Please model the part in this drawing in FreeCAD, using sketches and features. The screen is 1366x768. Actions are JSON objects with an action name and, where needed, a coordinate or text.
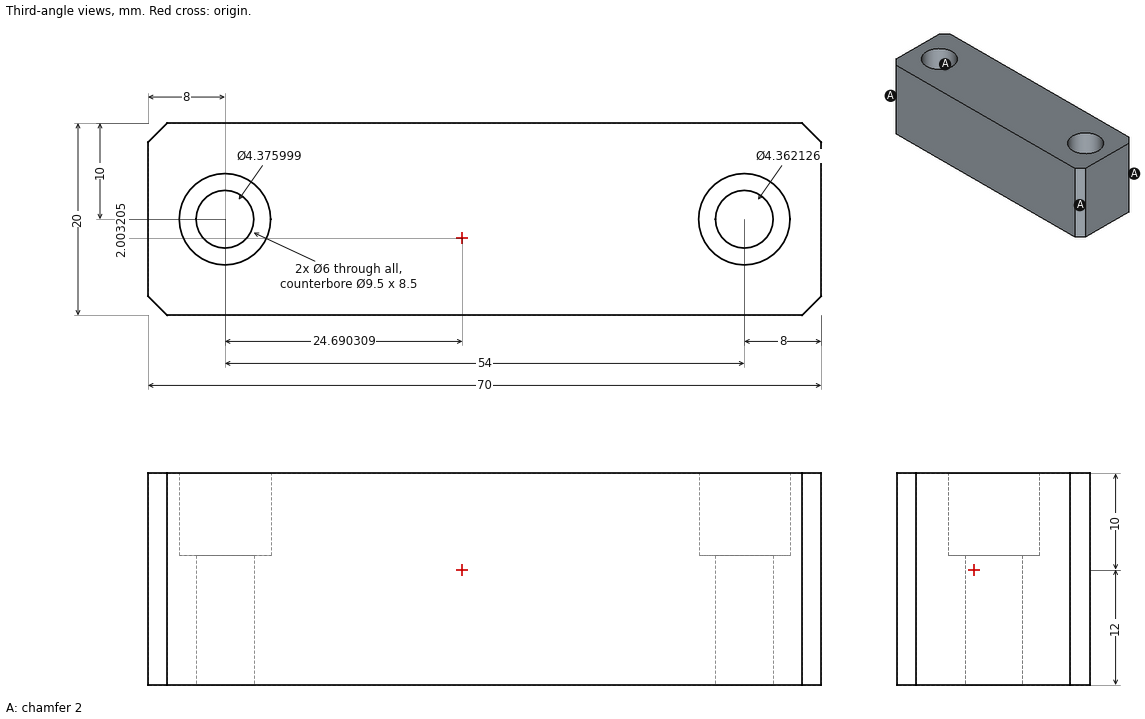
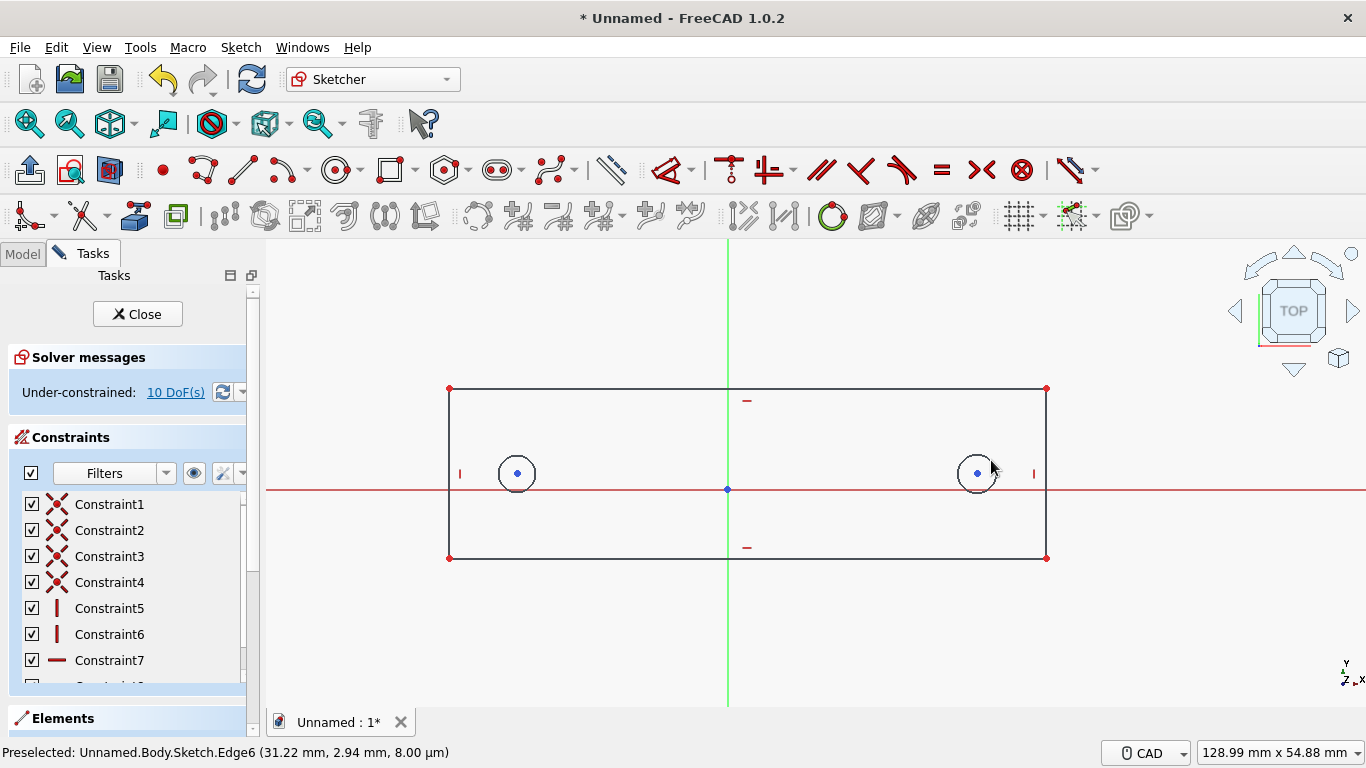
{"action": "left_click", "coordinate": [517, 474]}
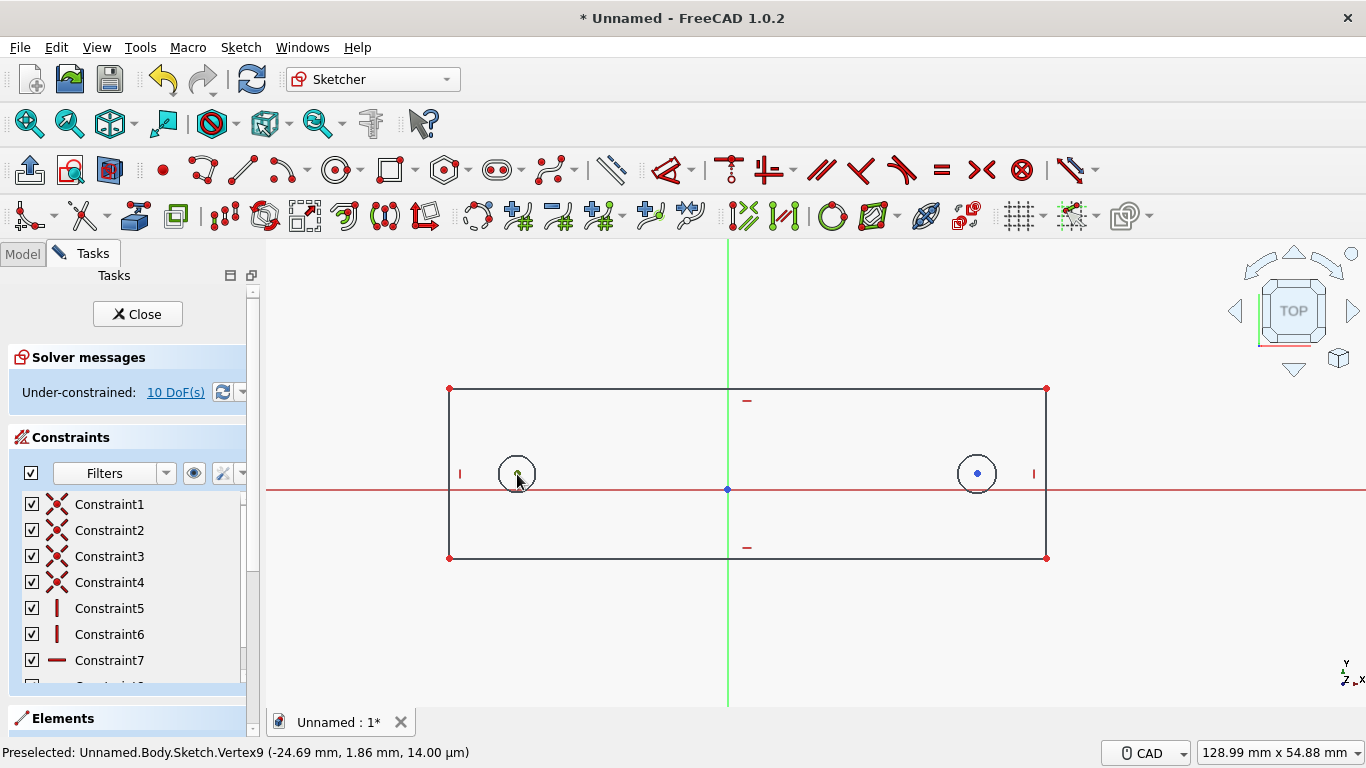
{"action": "left_click", "coordinate": [977, 474]}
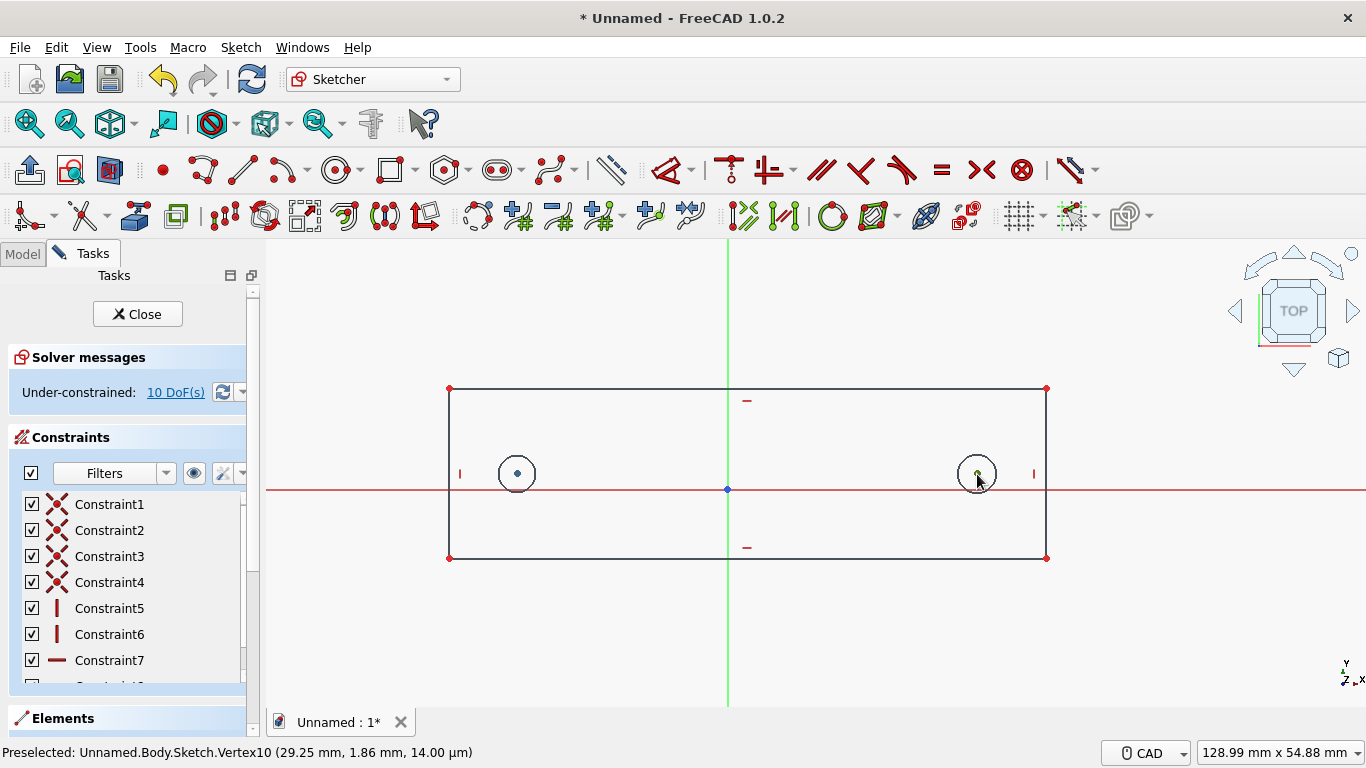
{"action": "key", "text": "h"}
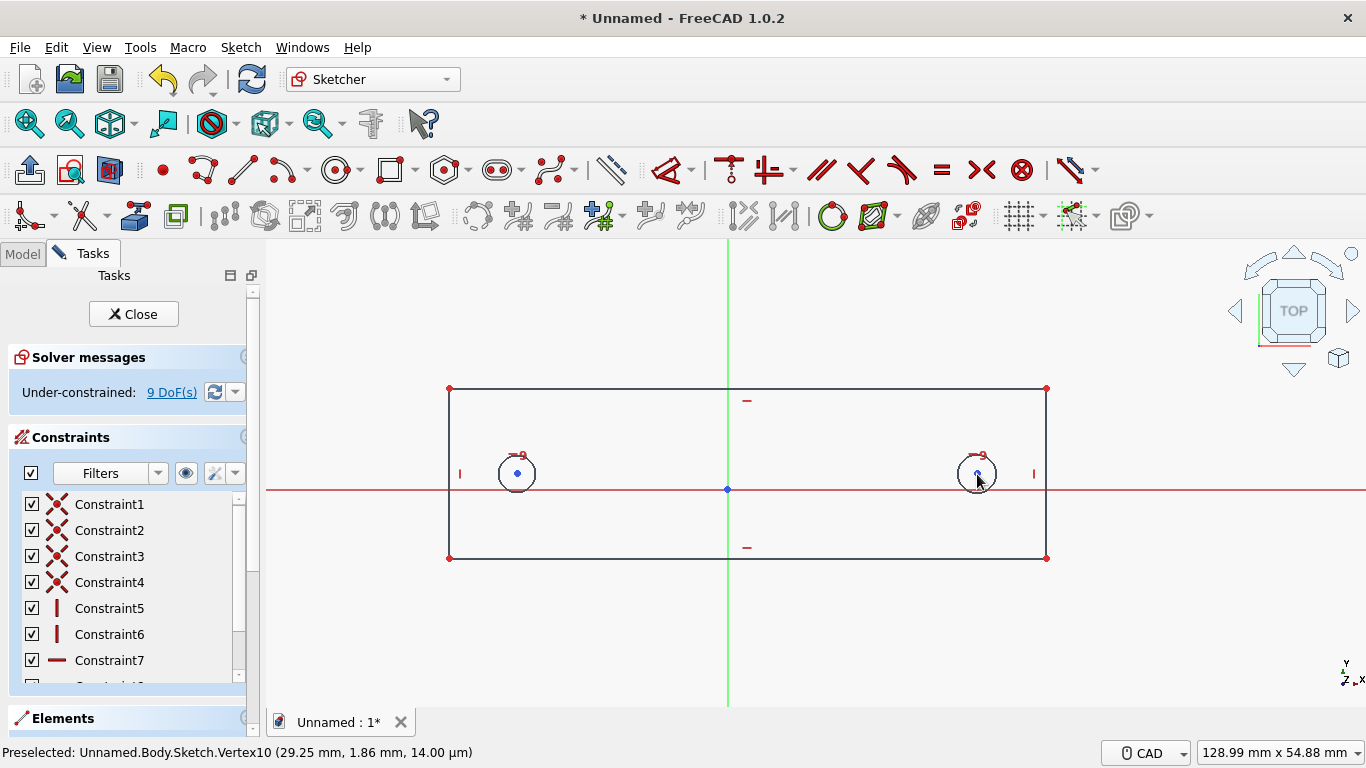
{"action": "left_click", "coordinate": [530, 461]}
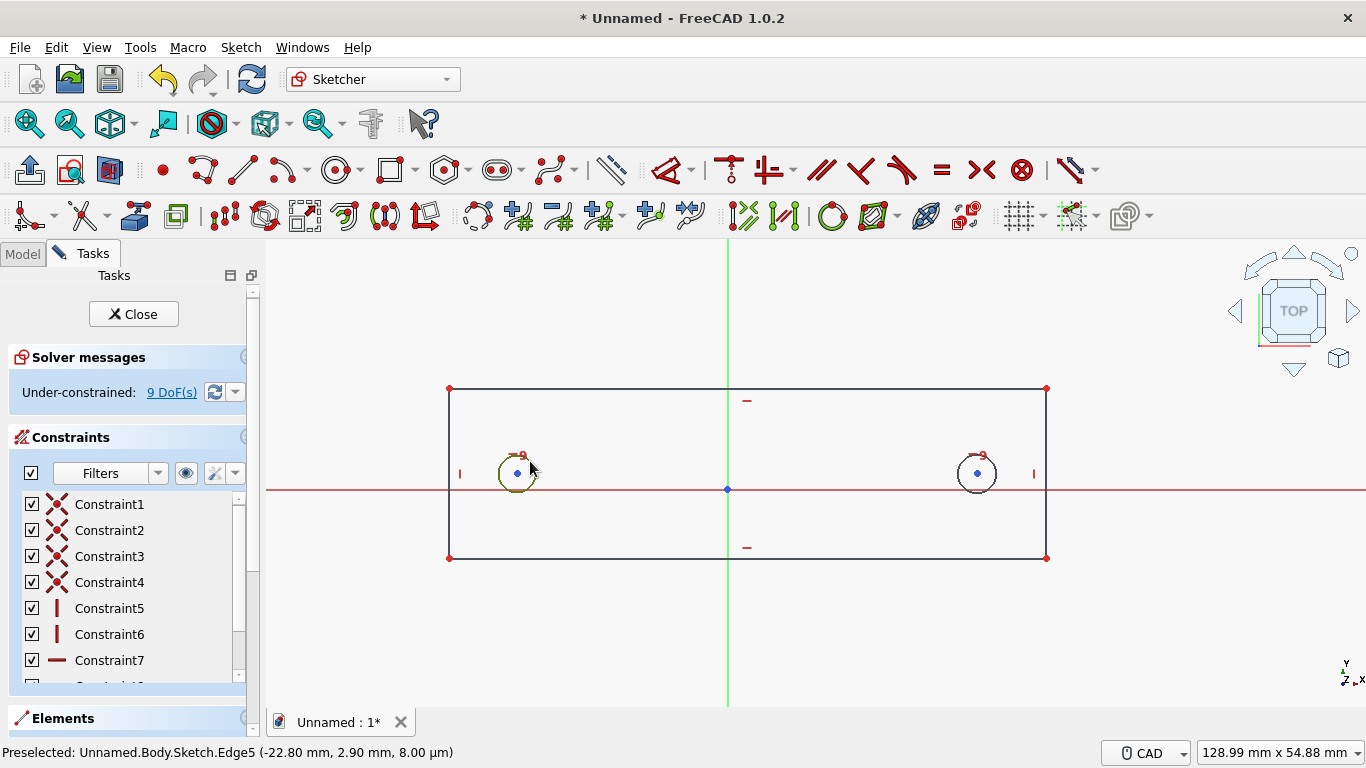
{"action": "key", "text": "k o"}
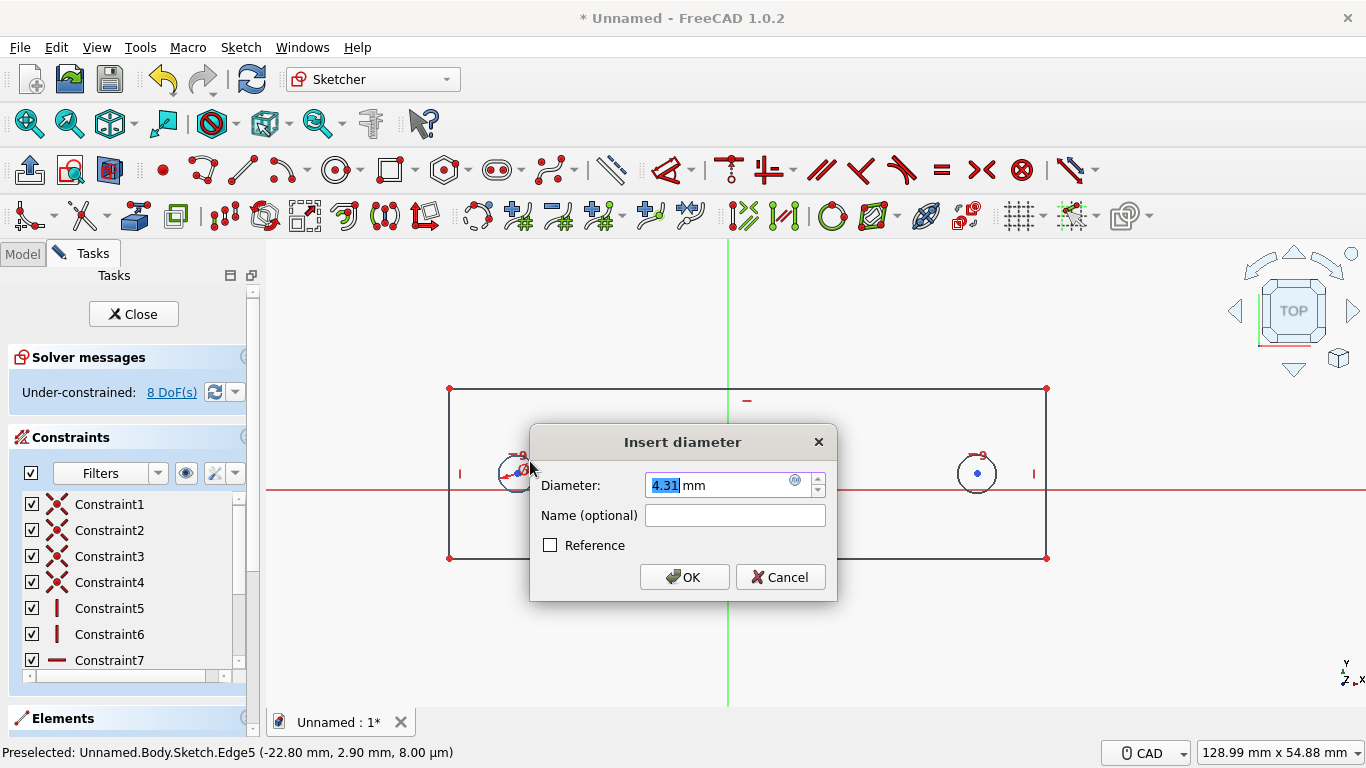
{"action": "type", "text": "4.375999"}
{"action": "key", "text": "Return"}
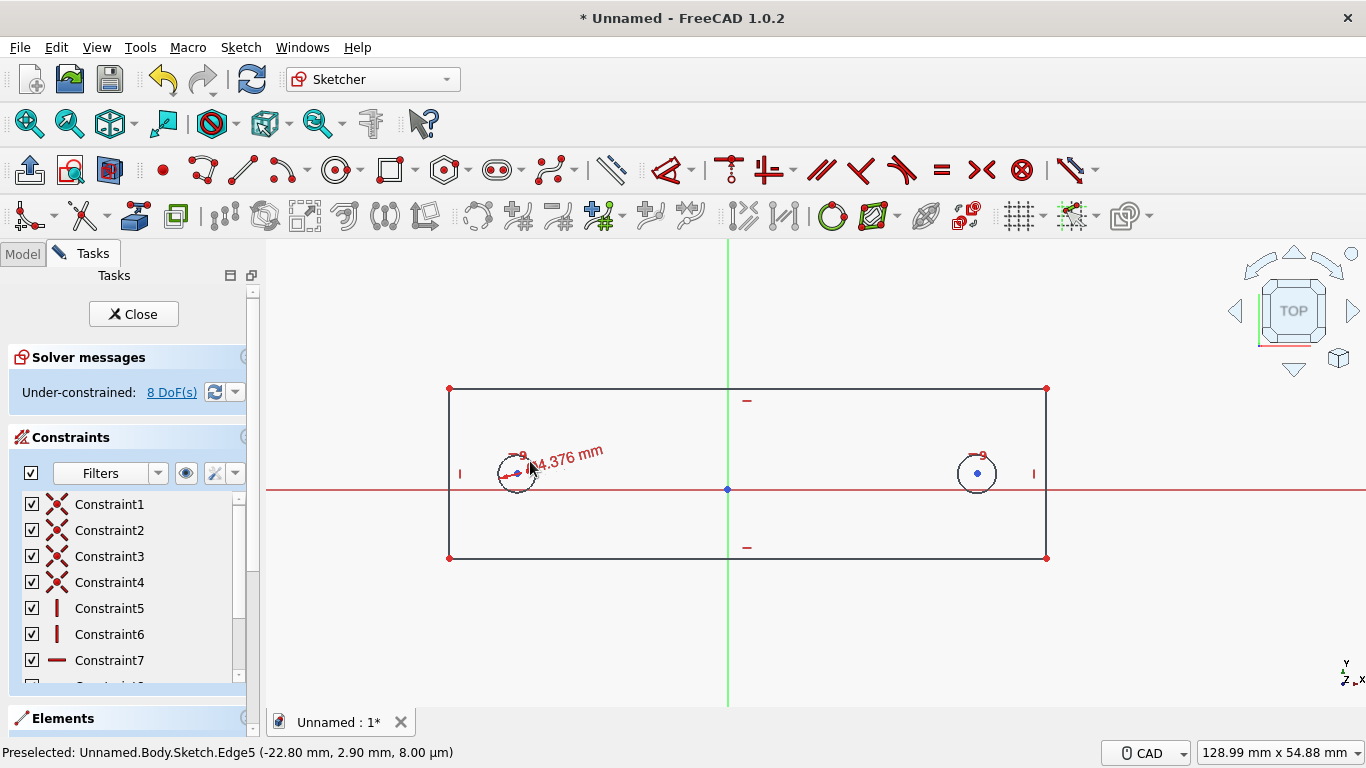
{"action": "left_click", "coordinate": [990, 460]}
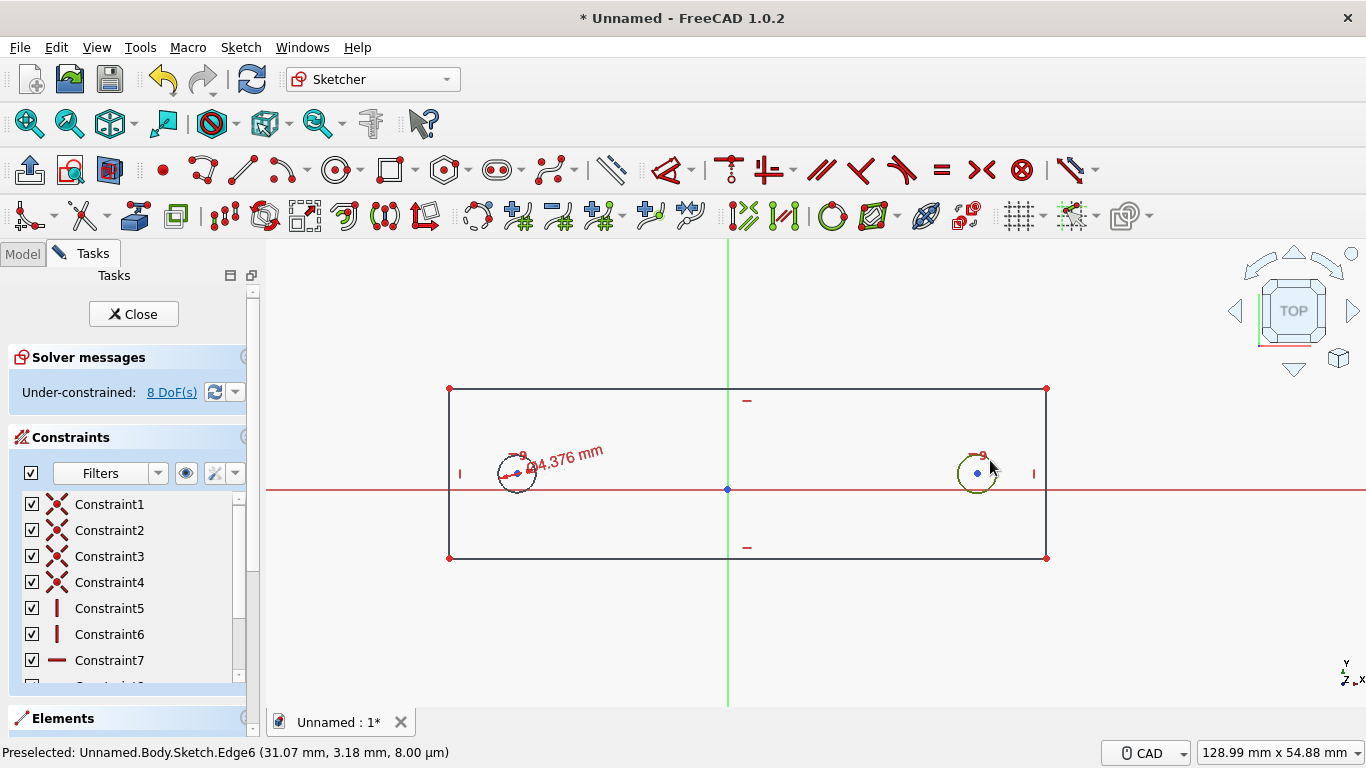
{"action": "key", "text": "k o"}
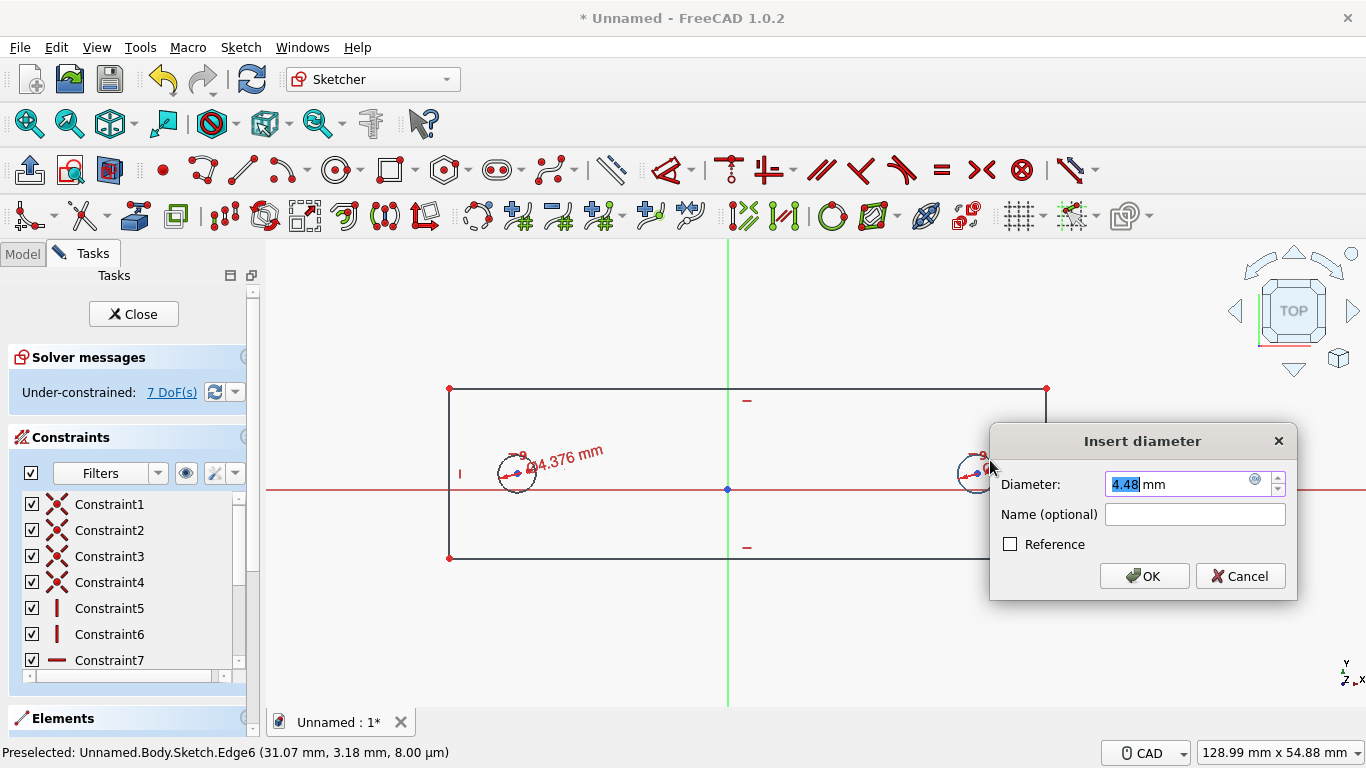
{"action": "type", "text": "4.362126"}
{"action": "key", "text": "Return"}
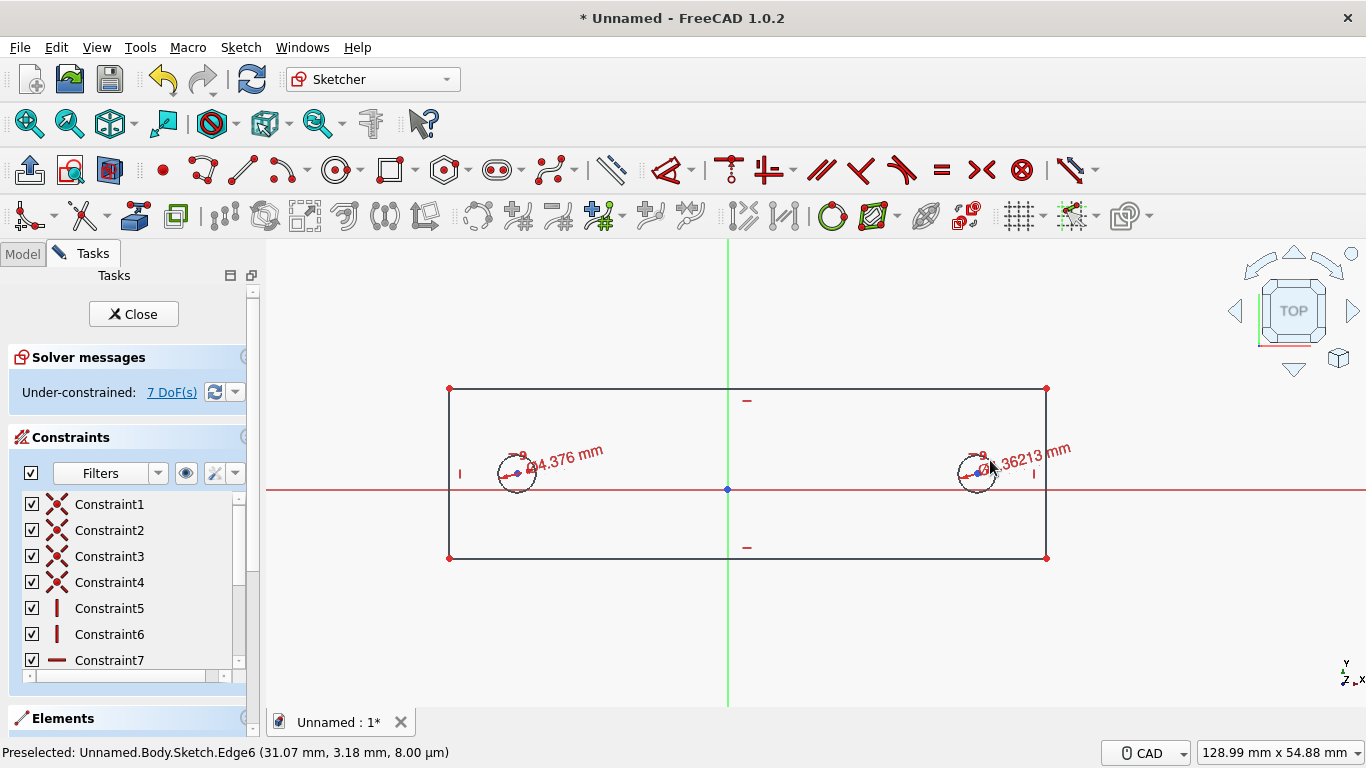
{"action": "left_click", "coordinate": [449, 440]}